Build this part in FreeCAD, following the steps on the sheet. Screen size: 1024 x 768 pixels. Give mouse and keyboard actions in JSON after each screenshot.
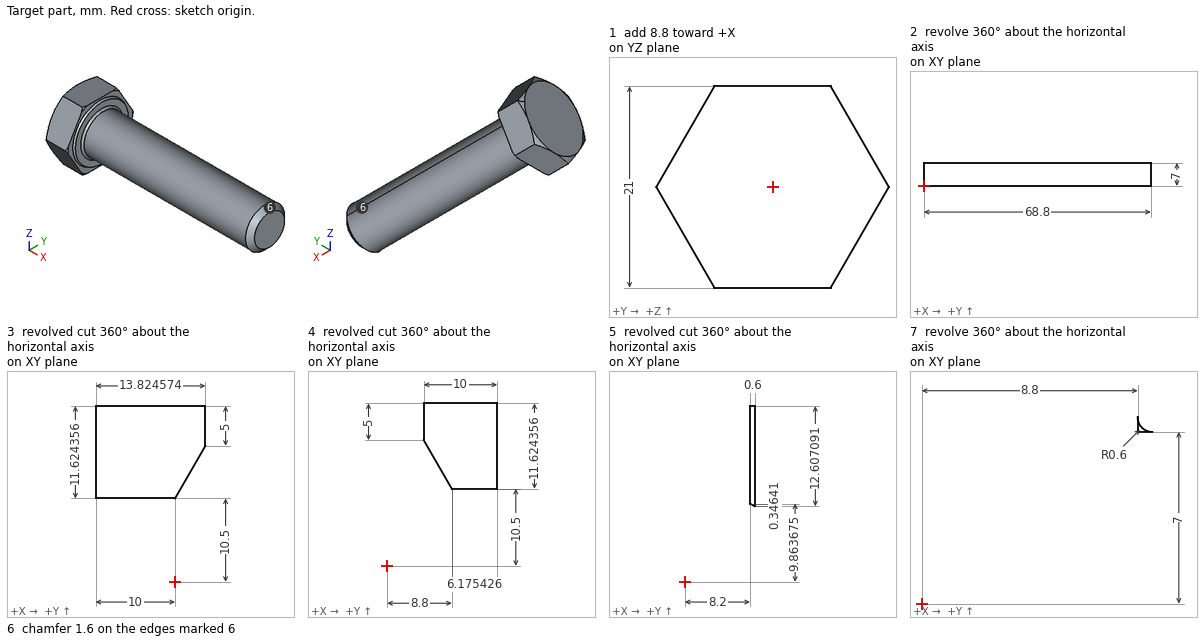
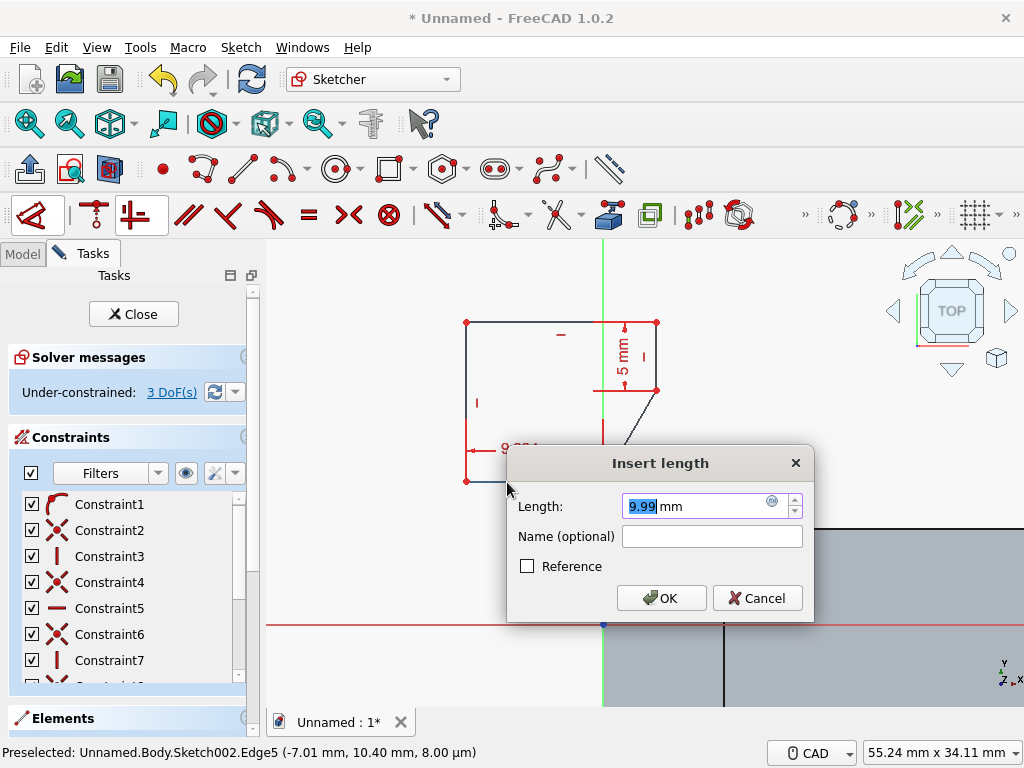
{"action": "type", "text": "10"}
{"action": "key", "text": "Return"}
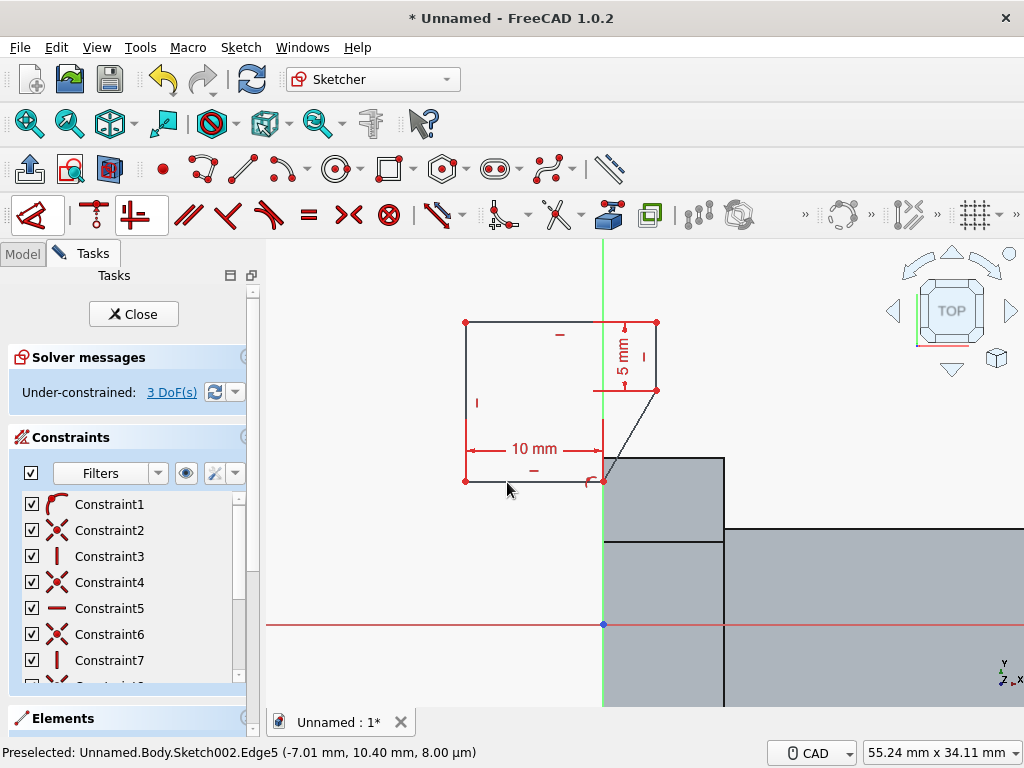
{"action": "left_click", "coordinate": [603, 482]}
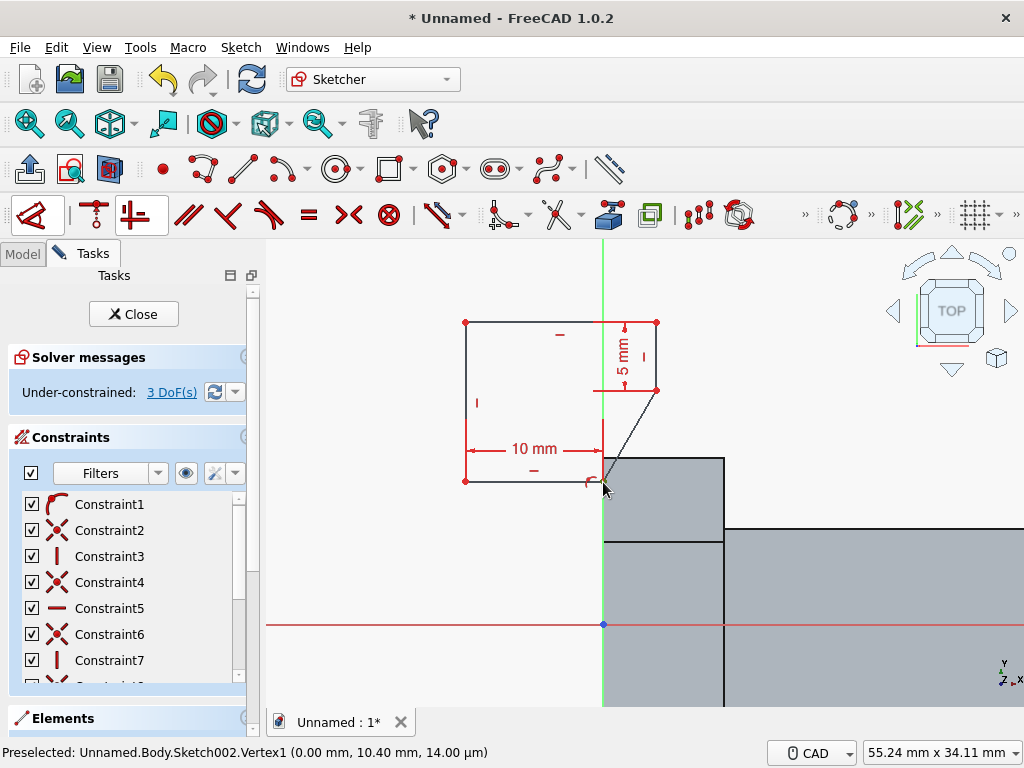
{"action": "left_click", "coordinate": [58, 216]}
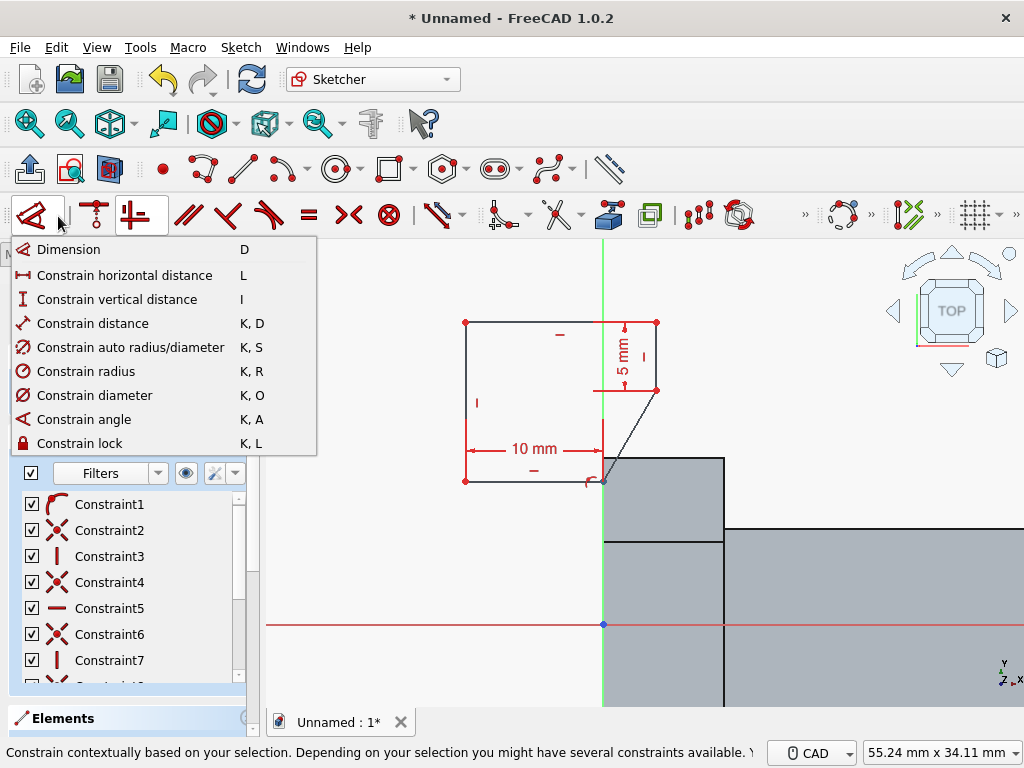
{"action": "left_click", "coordinate": [164, 299]}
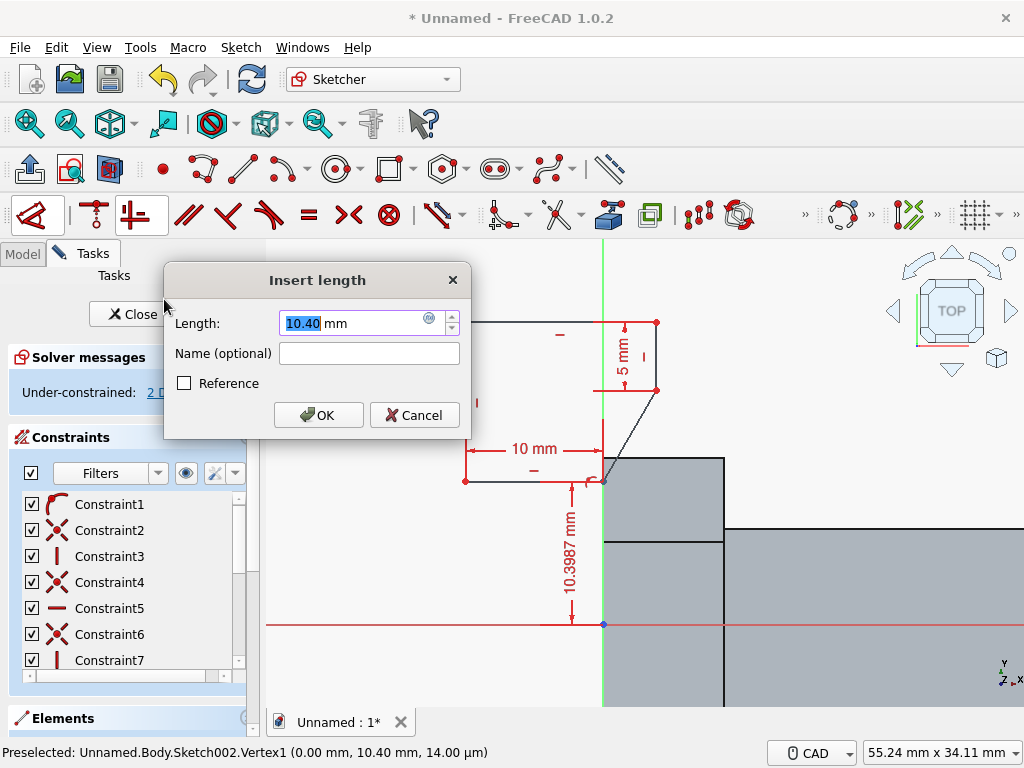
{"action": "type", "text": "10.5"}
{"action": "key", "text": "Return"}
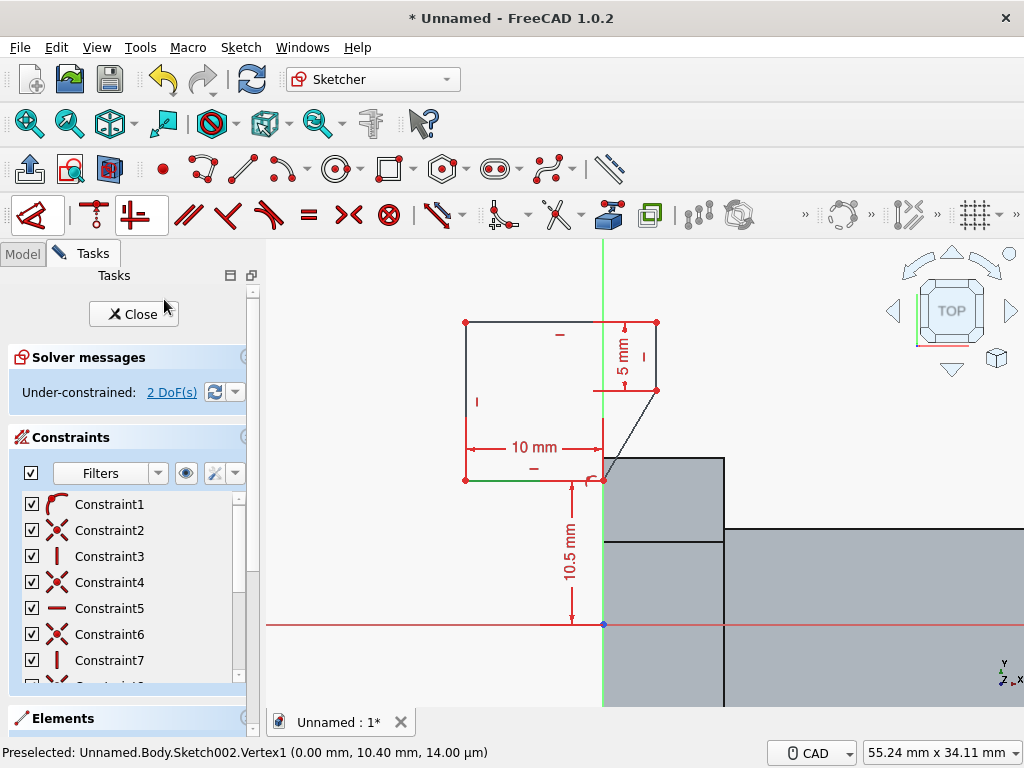
{"action": "left_click", "coordinate": [523, 322]}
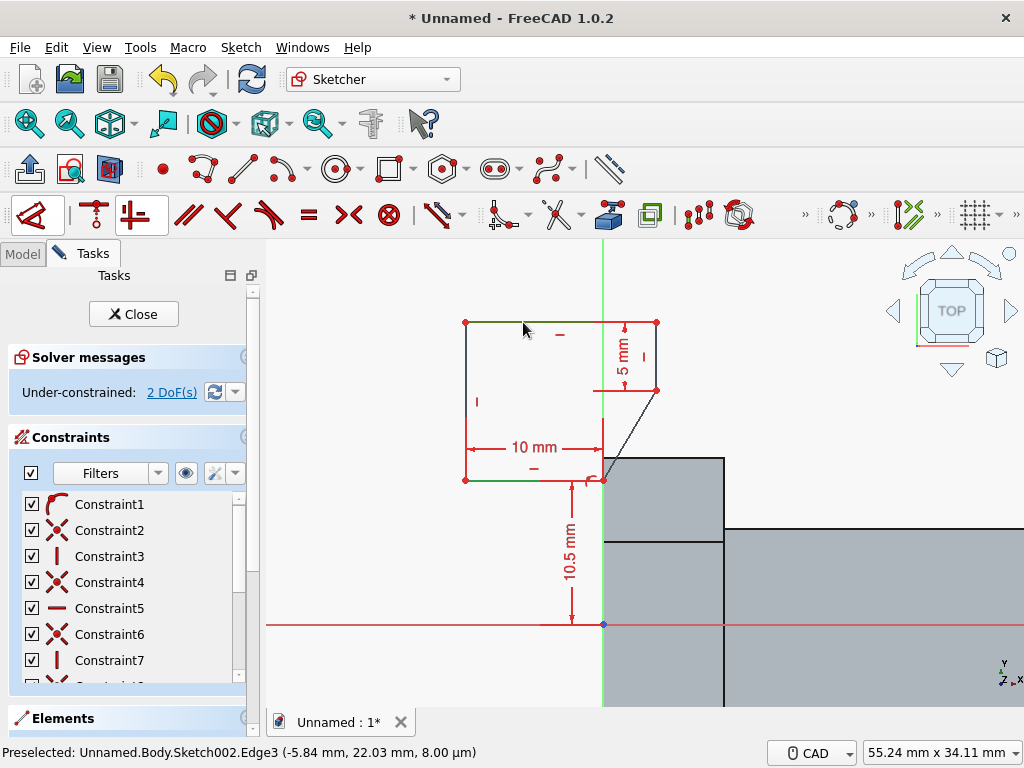
{"action": "left_click", "coordinate": [58, 216]}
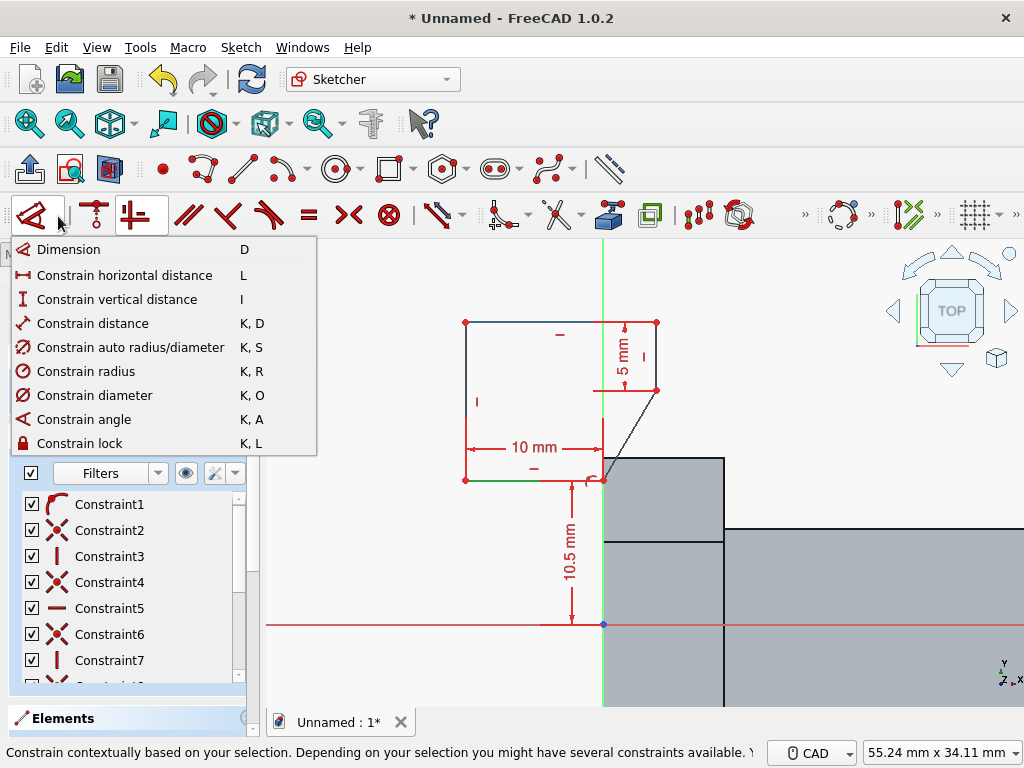
{"action": "left_click", "coordinate": [164, 275]}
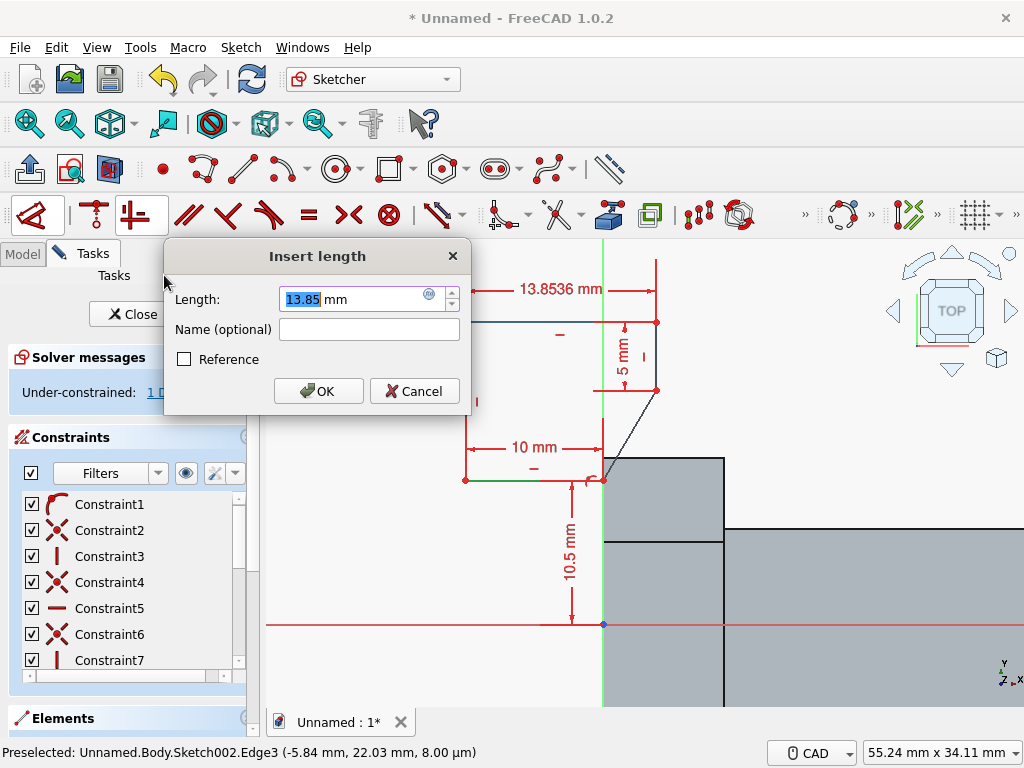
{"action": "type", "text": "13.824574"}
{"action": "key", "text": "Return"}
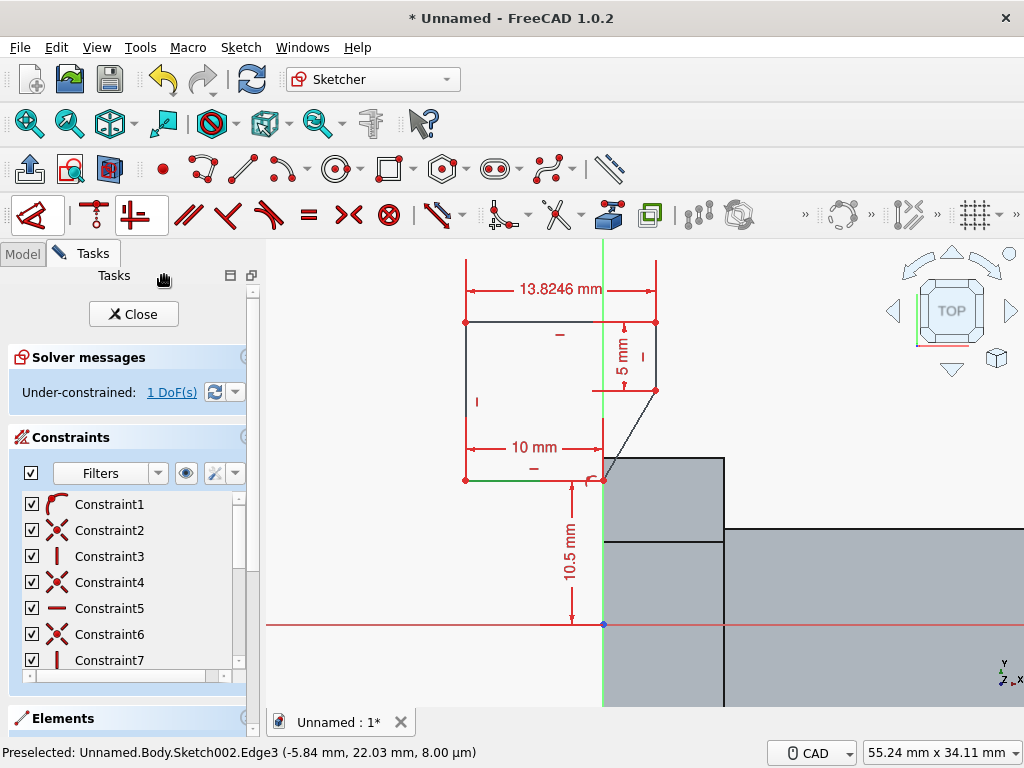
{"action": "left_click", "coordinate": [466, 370]}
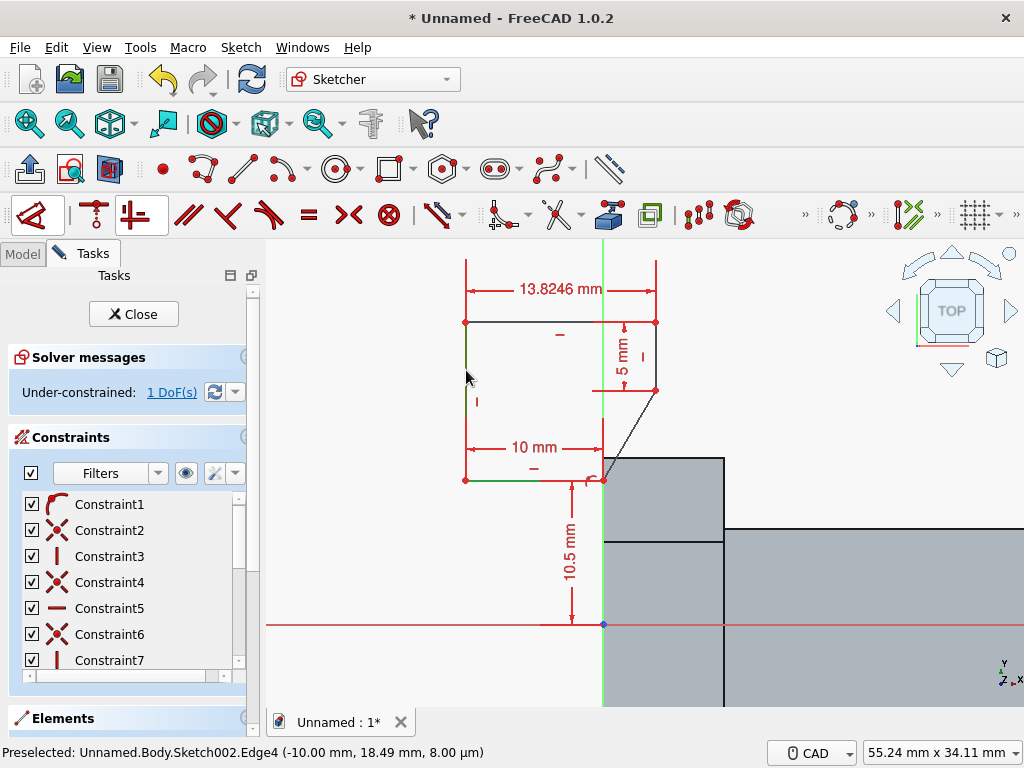
{"action": "key", "text": "i"}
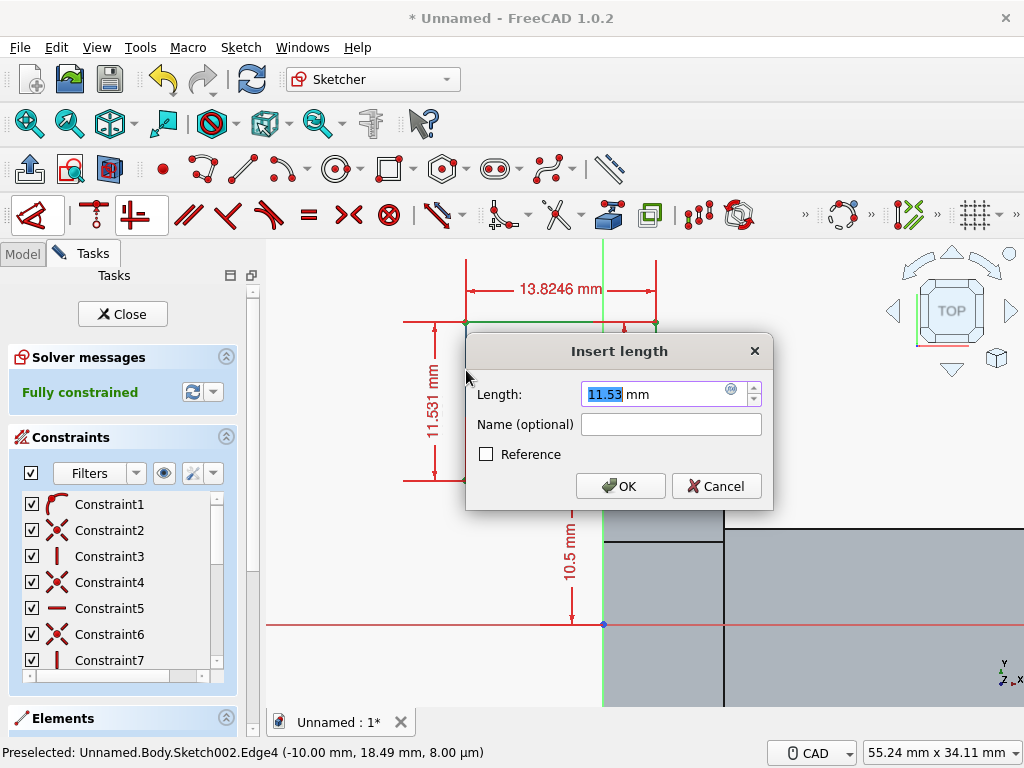
{"action": "type", "text": "11.624356"}
{"action": "key", "text": "Return"}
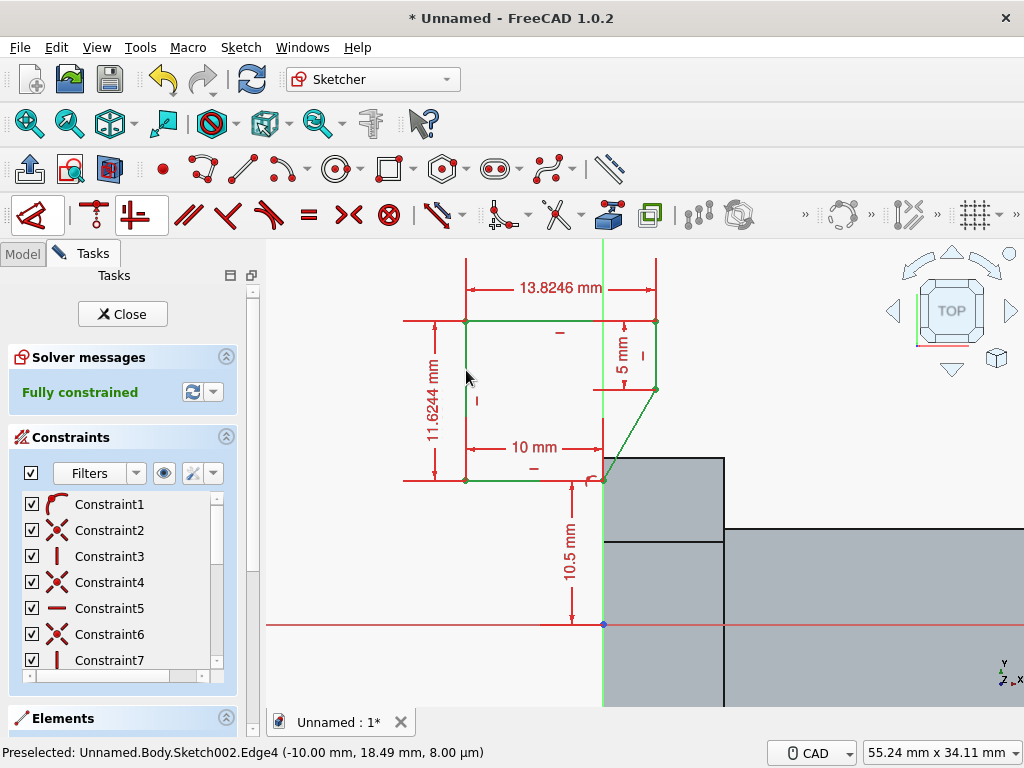
{"action": "left_click", "coordinate": [123, 314]}